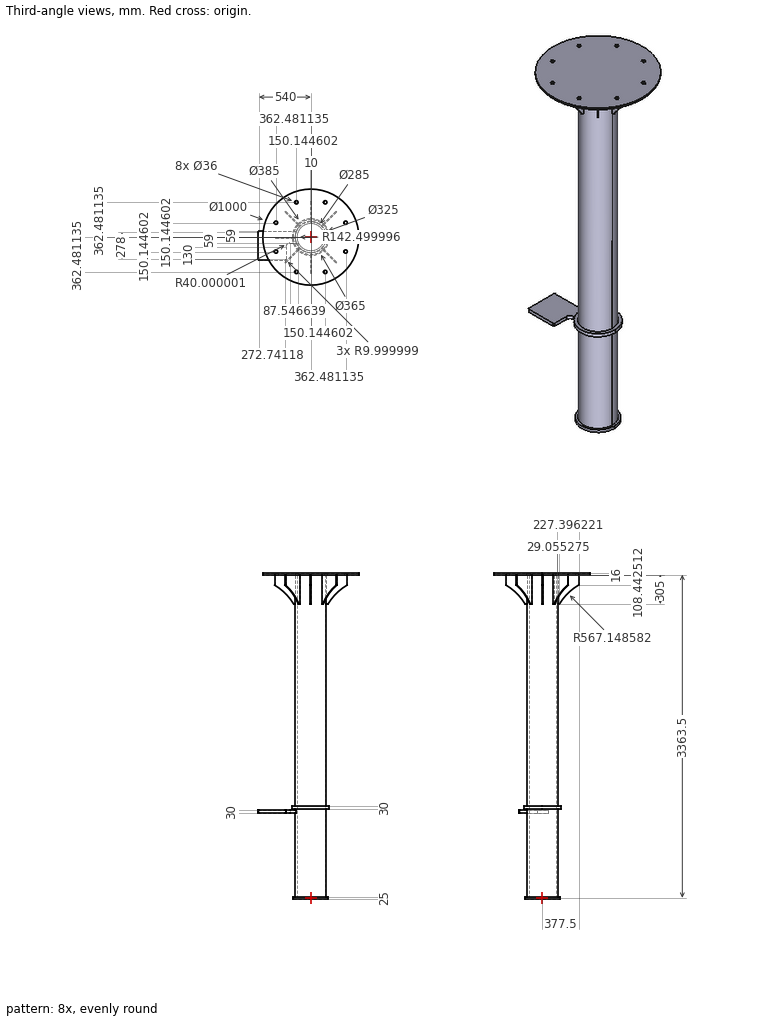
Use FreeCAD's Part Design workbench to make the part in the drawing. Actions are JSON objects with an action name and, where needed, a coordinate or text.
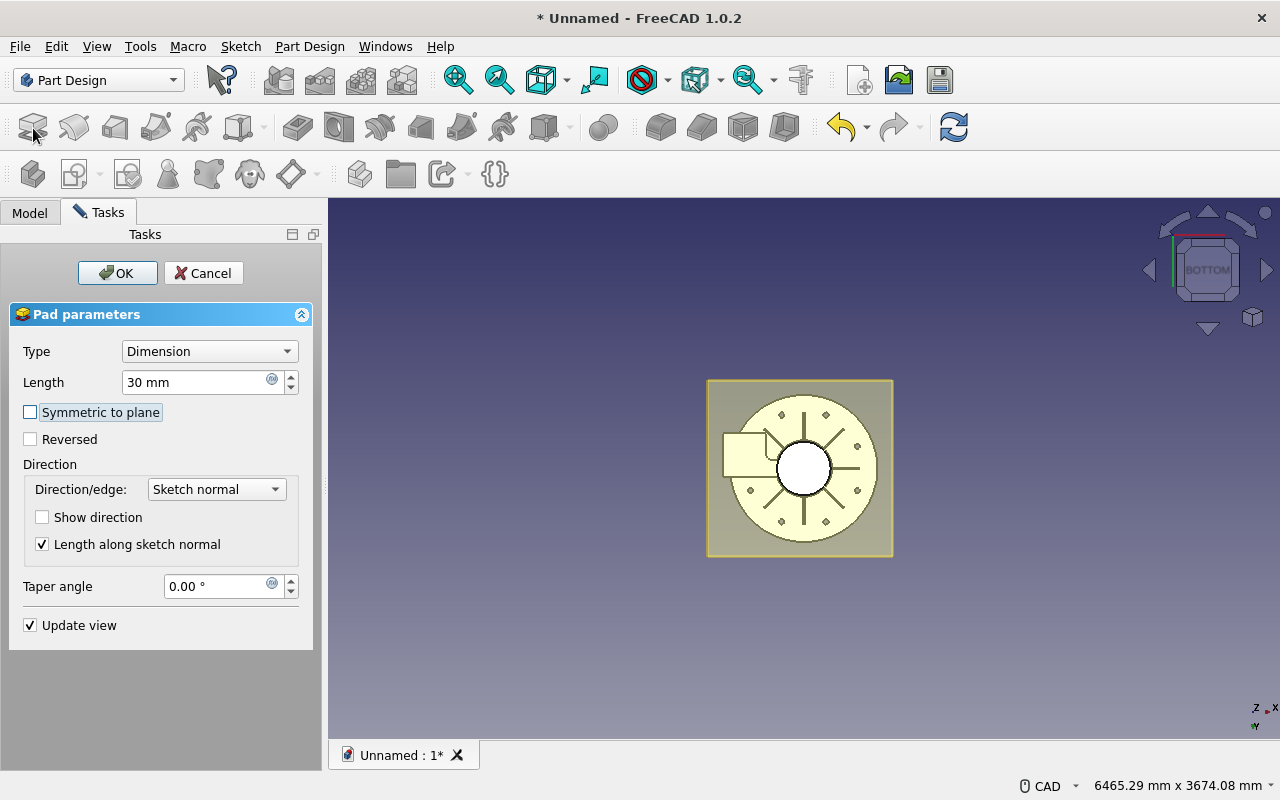
{"action": "left_click", "coordinate": [118, 273]}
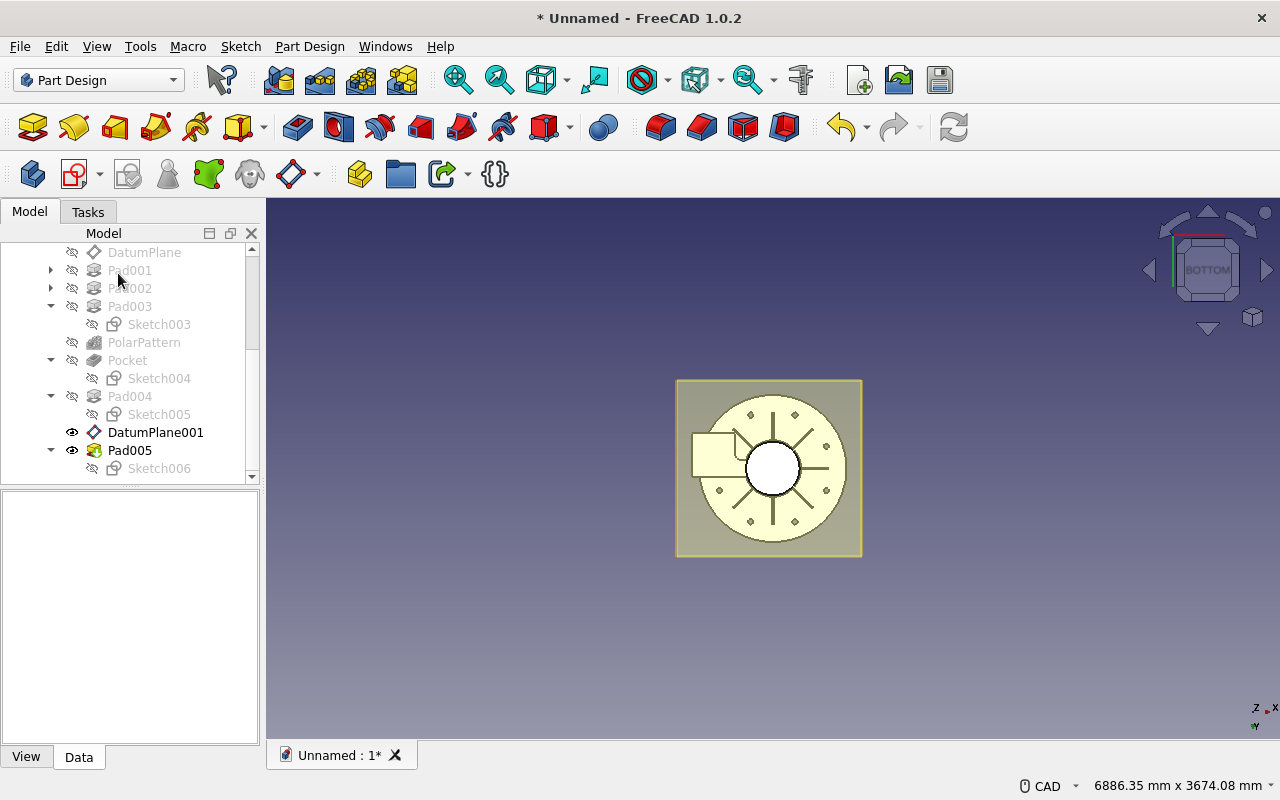
{"action": "left_click", "coordinate": [117, 432]}
{"action": "key", "text": "space"}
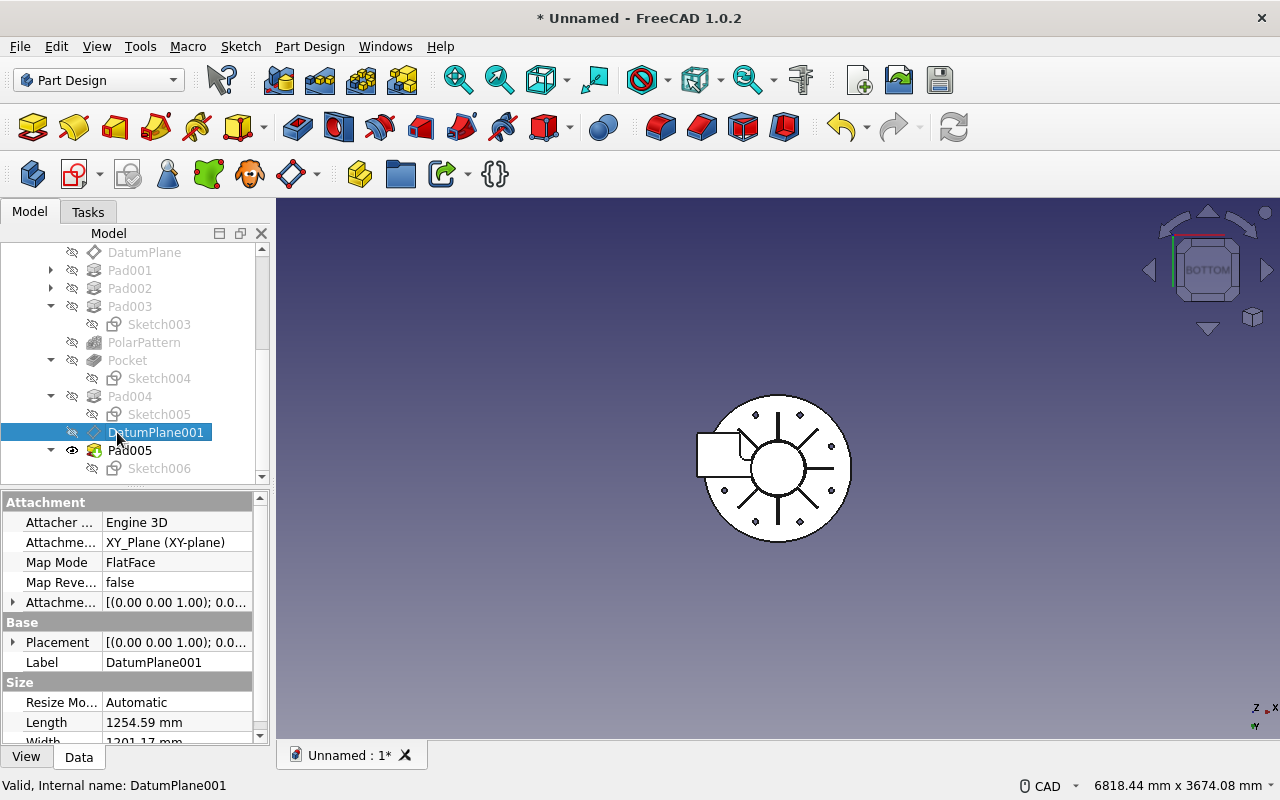
{"action": "key", "text": "0"}